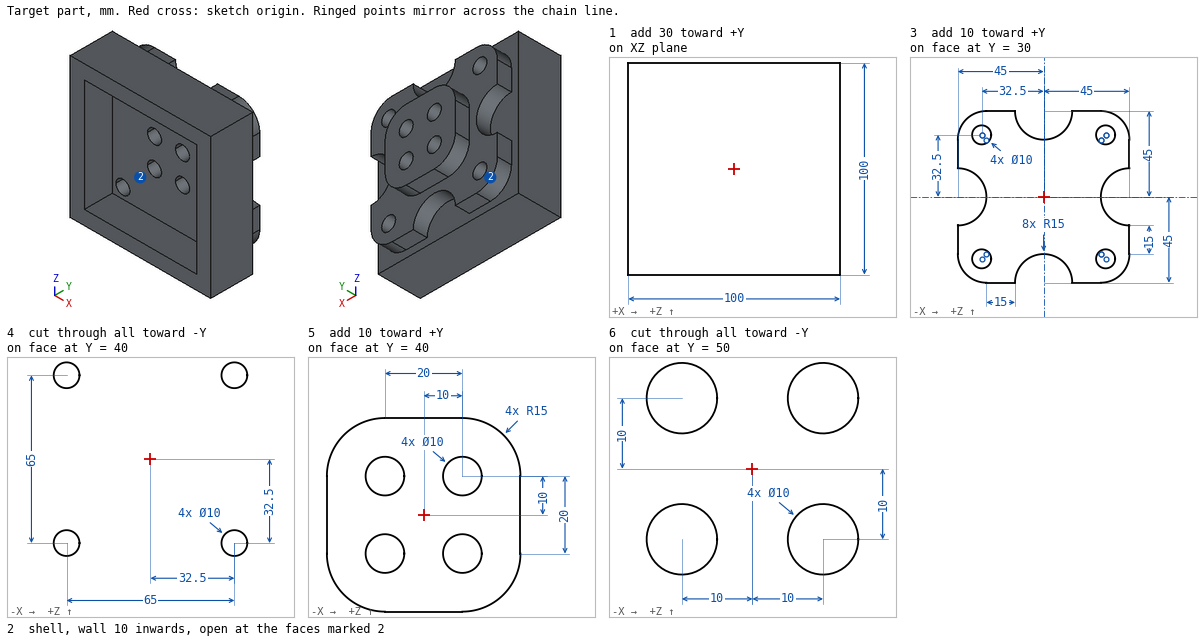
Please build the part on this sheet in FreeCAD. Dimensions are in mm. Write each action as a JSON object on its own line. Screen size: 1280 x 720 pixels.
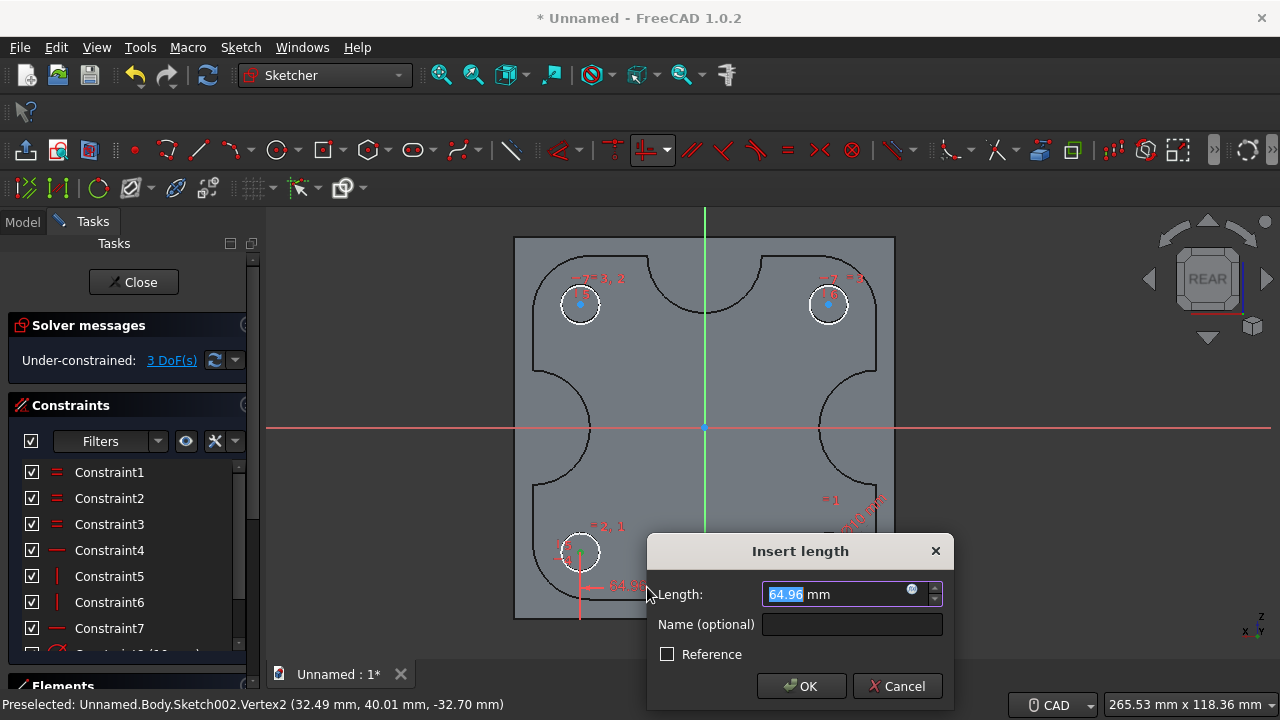
{"action": "type", "text": "65"}
{"action": "key", "text": "Return"}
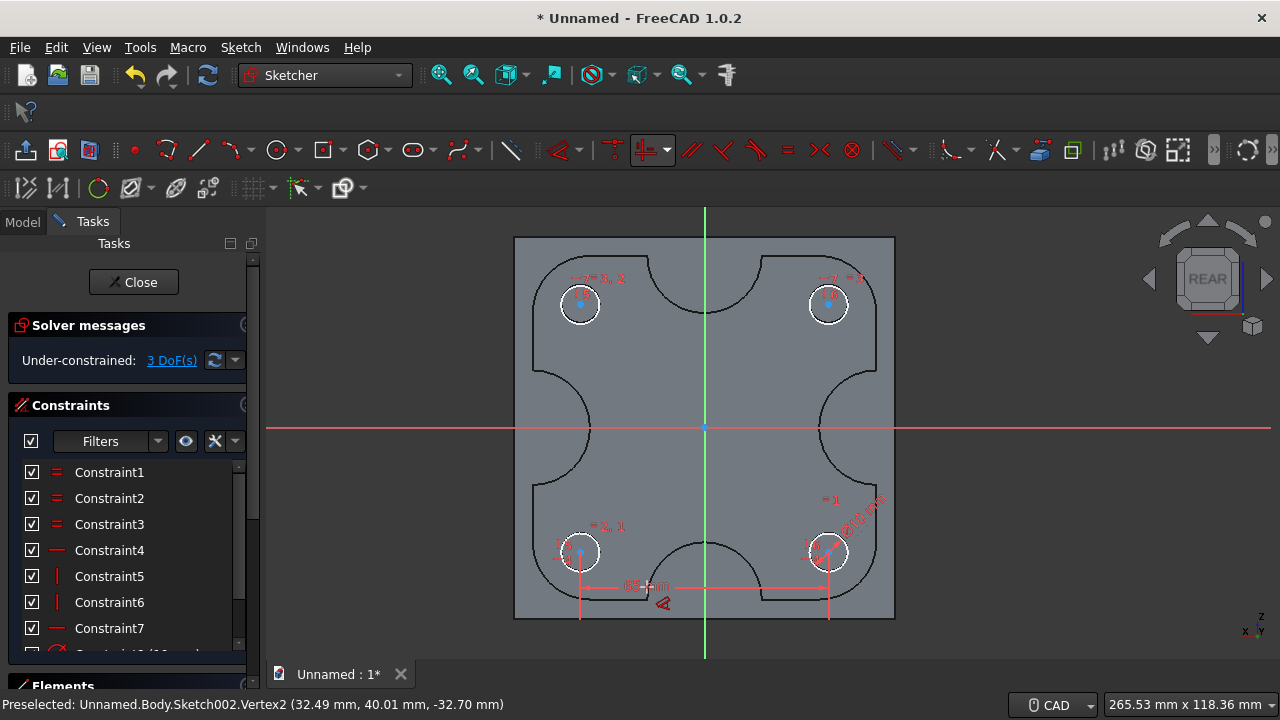
{"action": "left_click", "coordinate": [580, 553]}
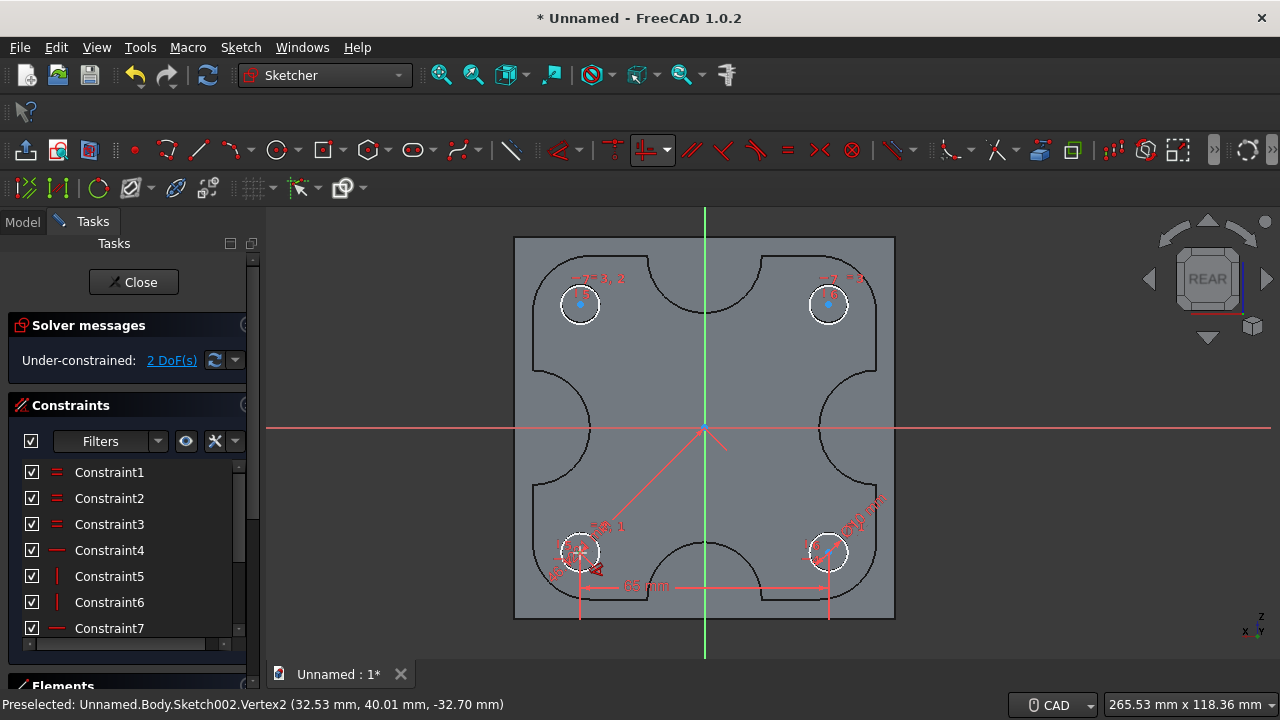
{"action": "left_click", "coordinate": [580, 305]}
{"action": "left_click", "coordinate": [546, 372]}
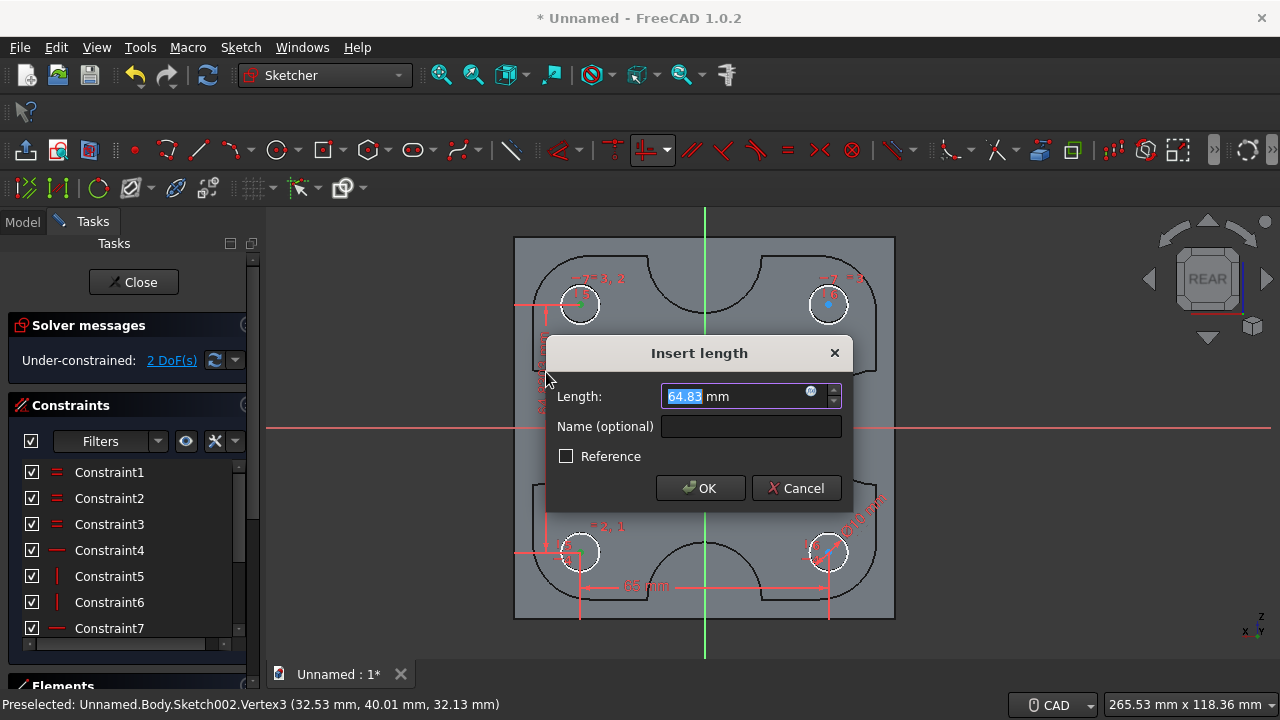
{"action": "type", "text": "65"}
{"action": "key", "text": "Return"}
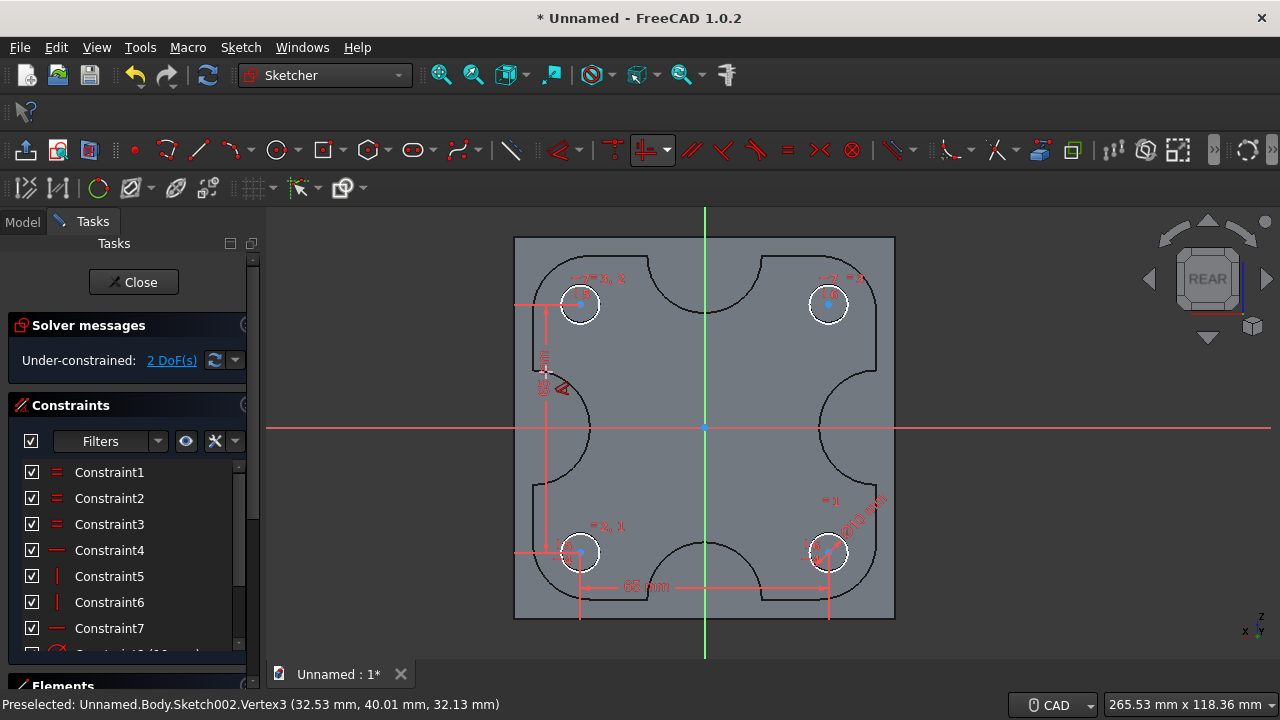
{"action": "left_click", "coordinate": [829, 553]}
{"action": "left_click", "coordinate": [767, 587]}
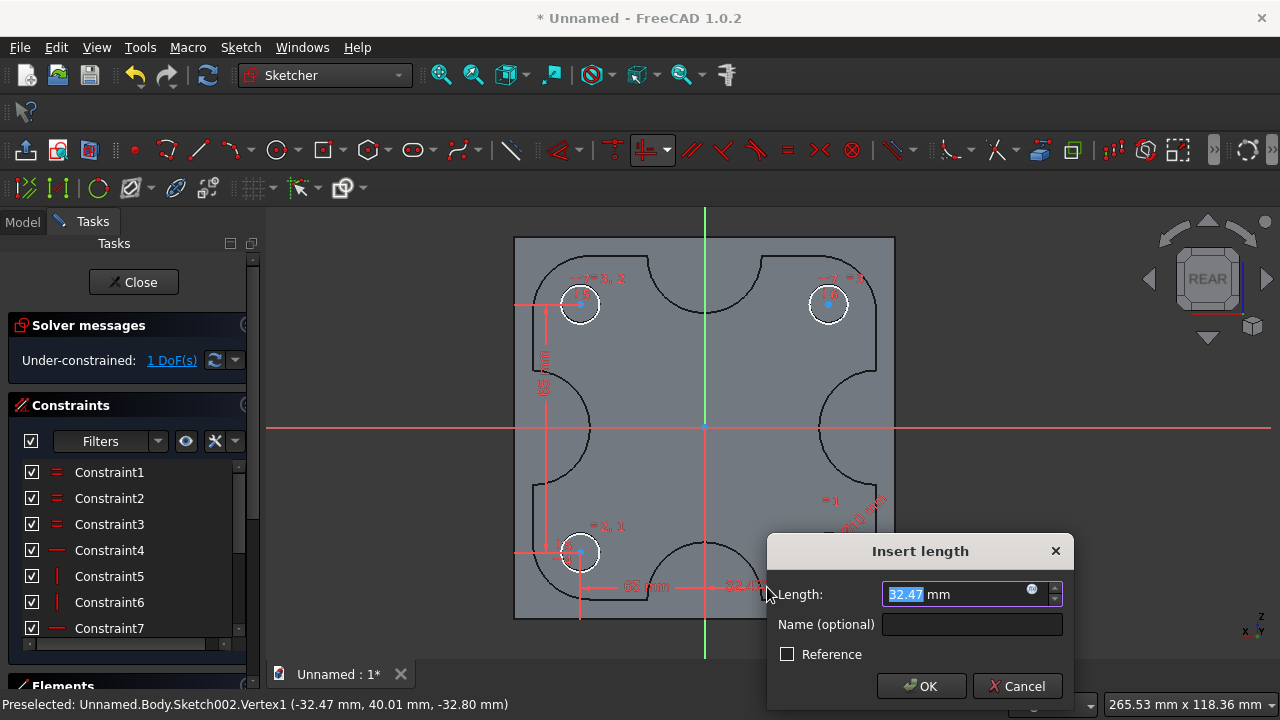
{"action": "type", "text": "32.5"}
{"action": "key", "text": "Return"}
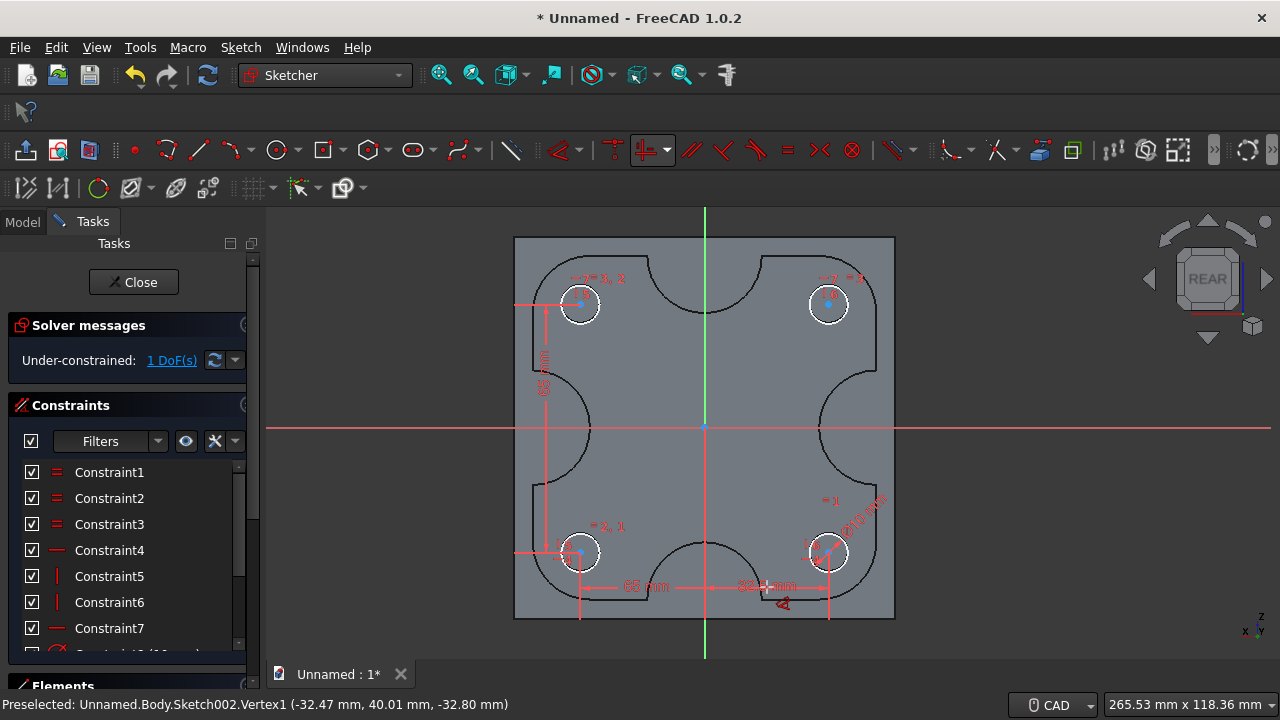
{"action": "left_click", "coordinate": [829, 553]}
{"action": "left_click", "coordinate": [863, 490]}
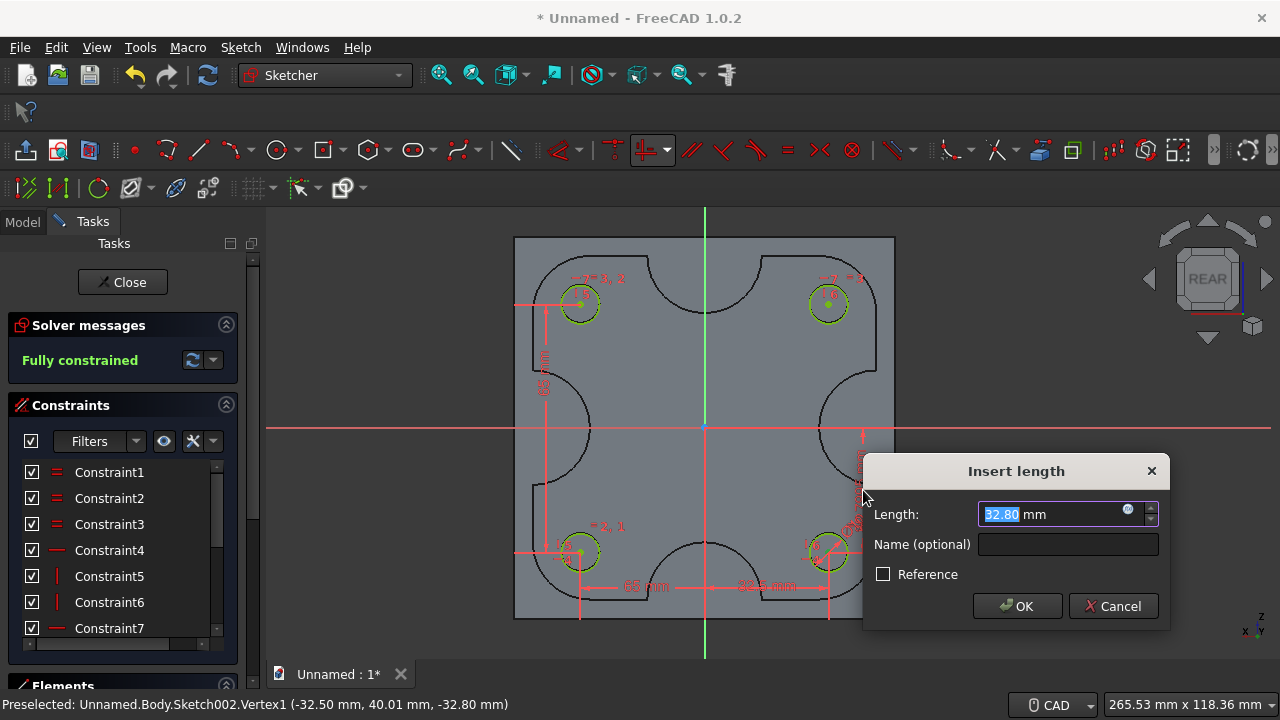
{"action": "type", "text": "32.5"}
{"action": "key", "text": "Return"}
{"action": "key", "text": "Escape"}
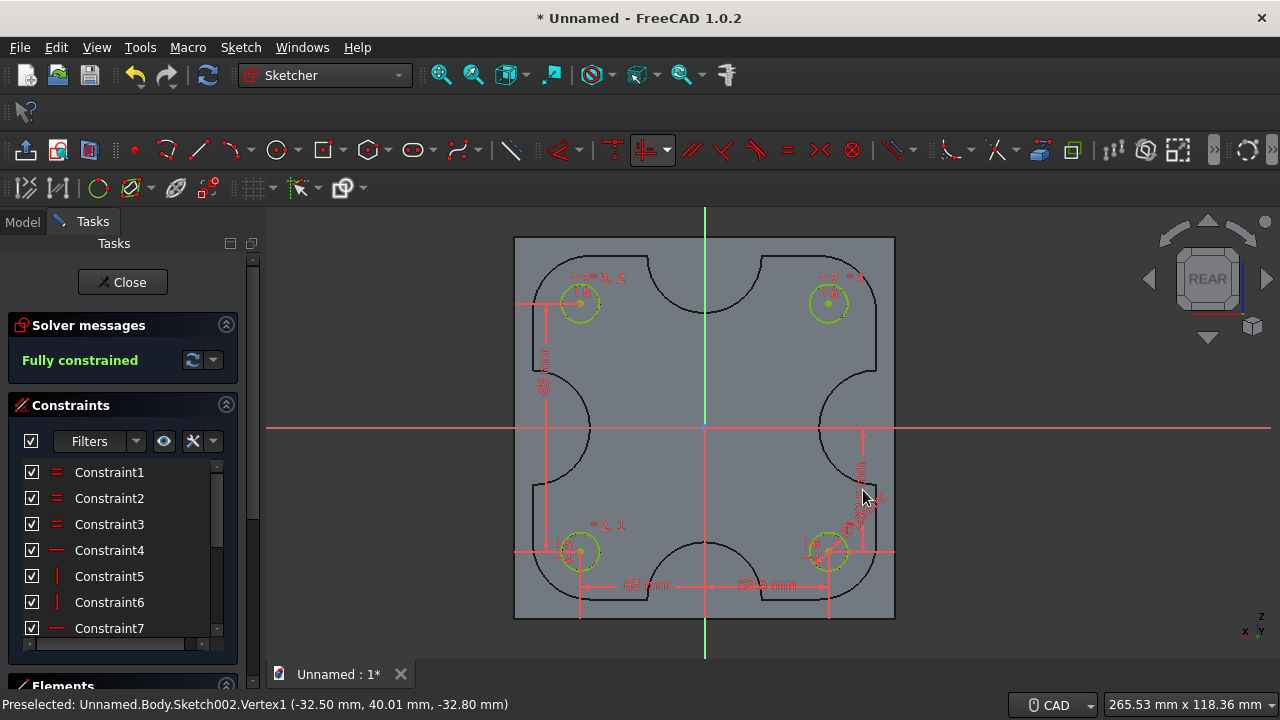
{"action": "left_click", "coordinate": [123, 282]}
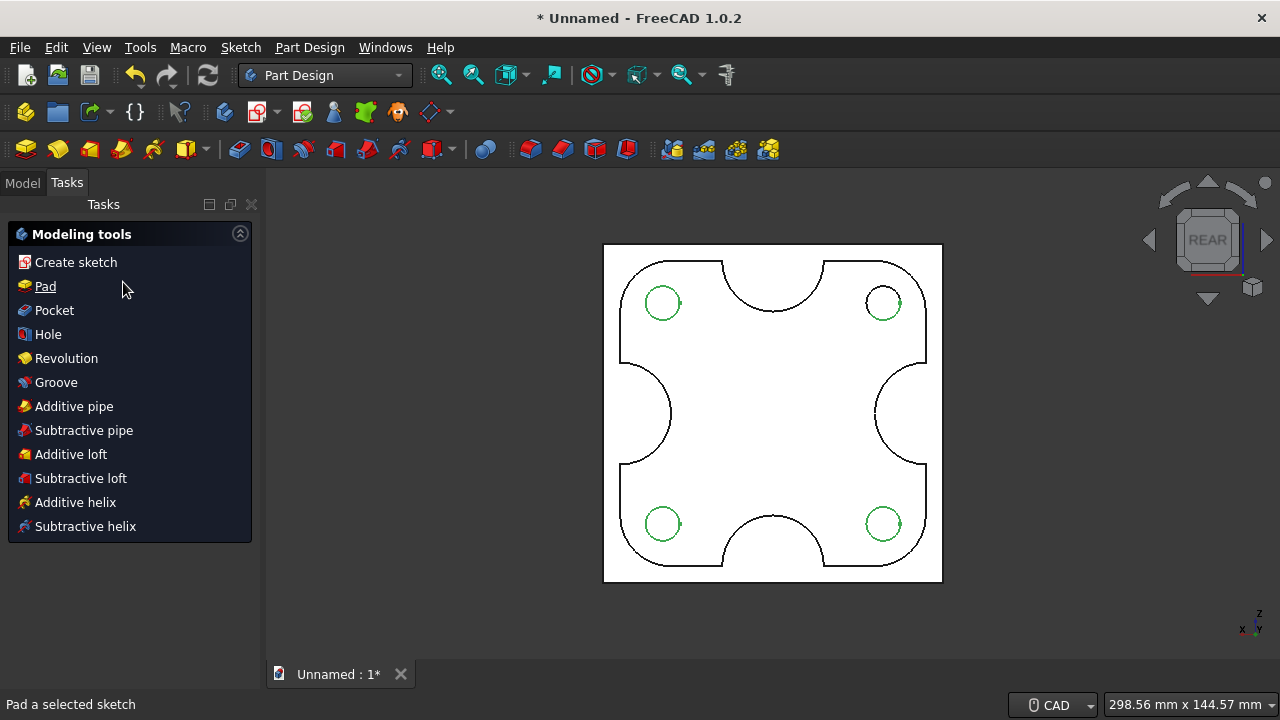
{"action": "left_click", "coordinate": [240, 150]}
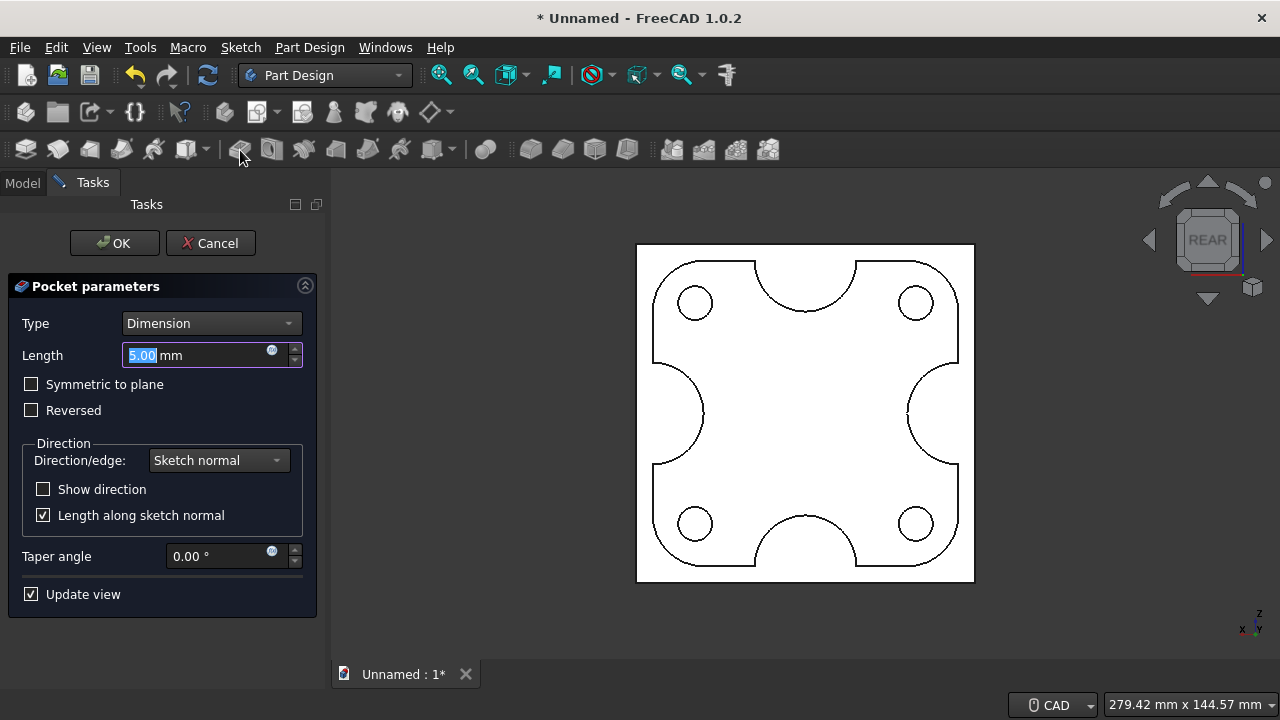
{"action": "left_click", "coordinate": [212, 324]}